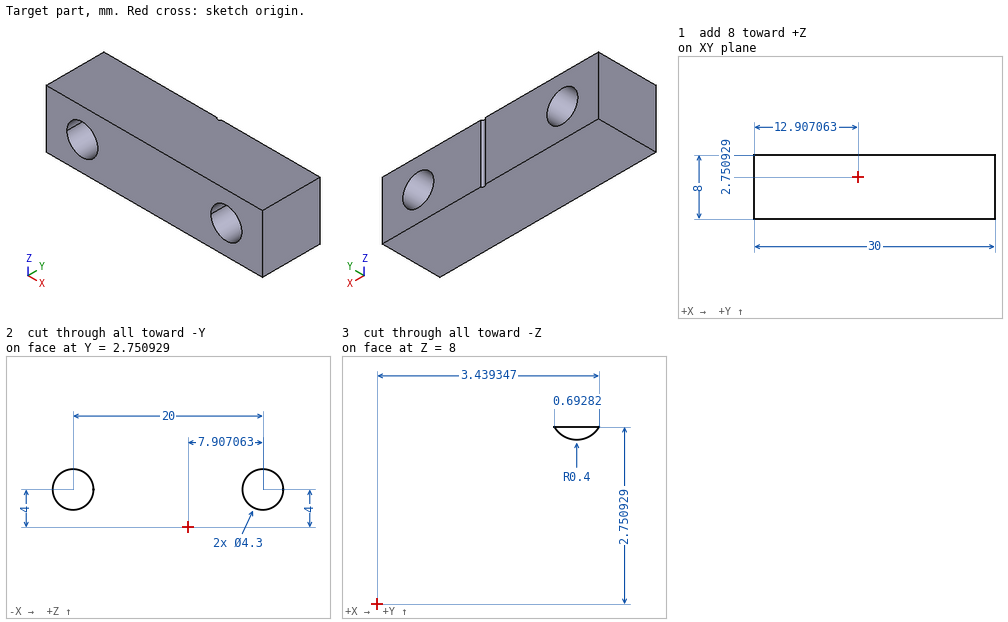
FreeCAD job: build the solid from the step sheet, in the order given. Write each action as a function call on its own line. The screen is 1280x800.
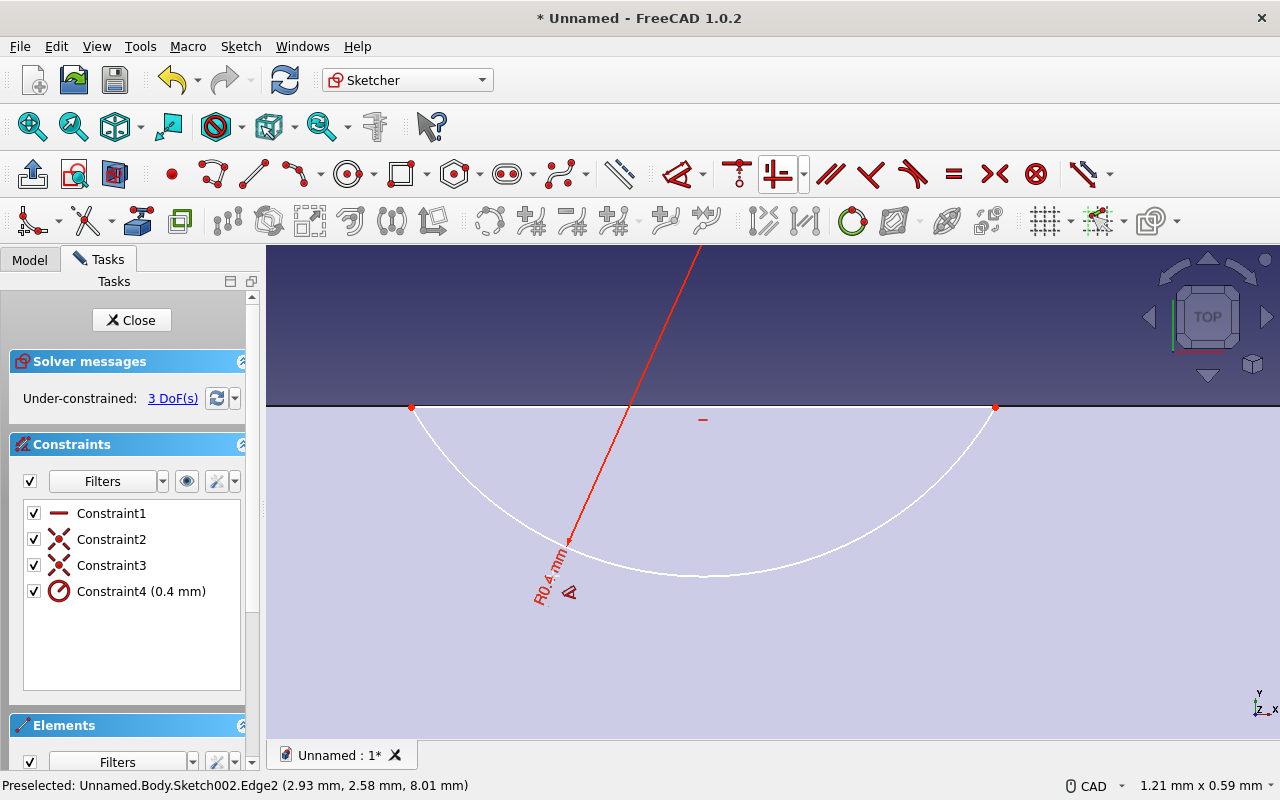
click(820, 407)
click(703, 373)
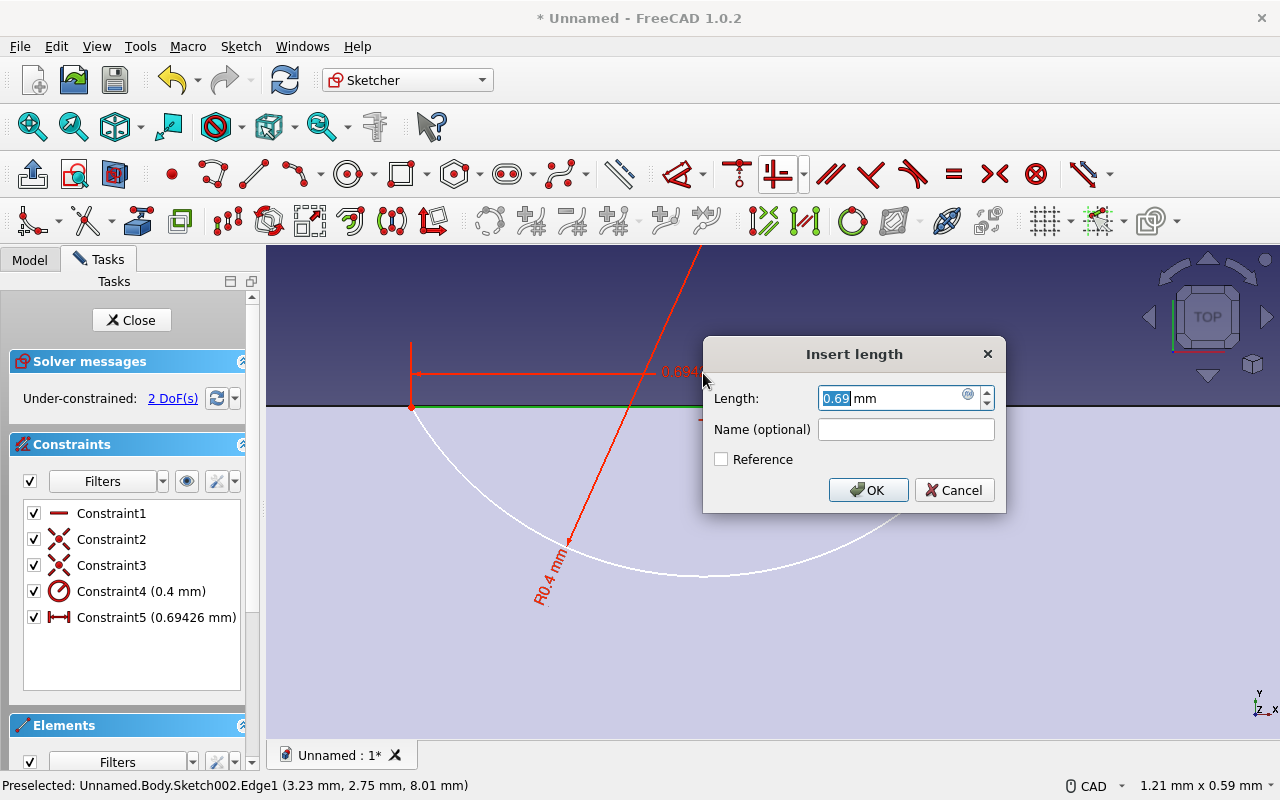
text(0.69282)
key(Return)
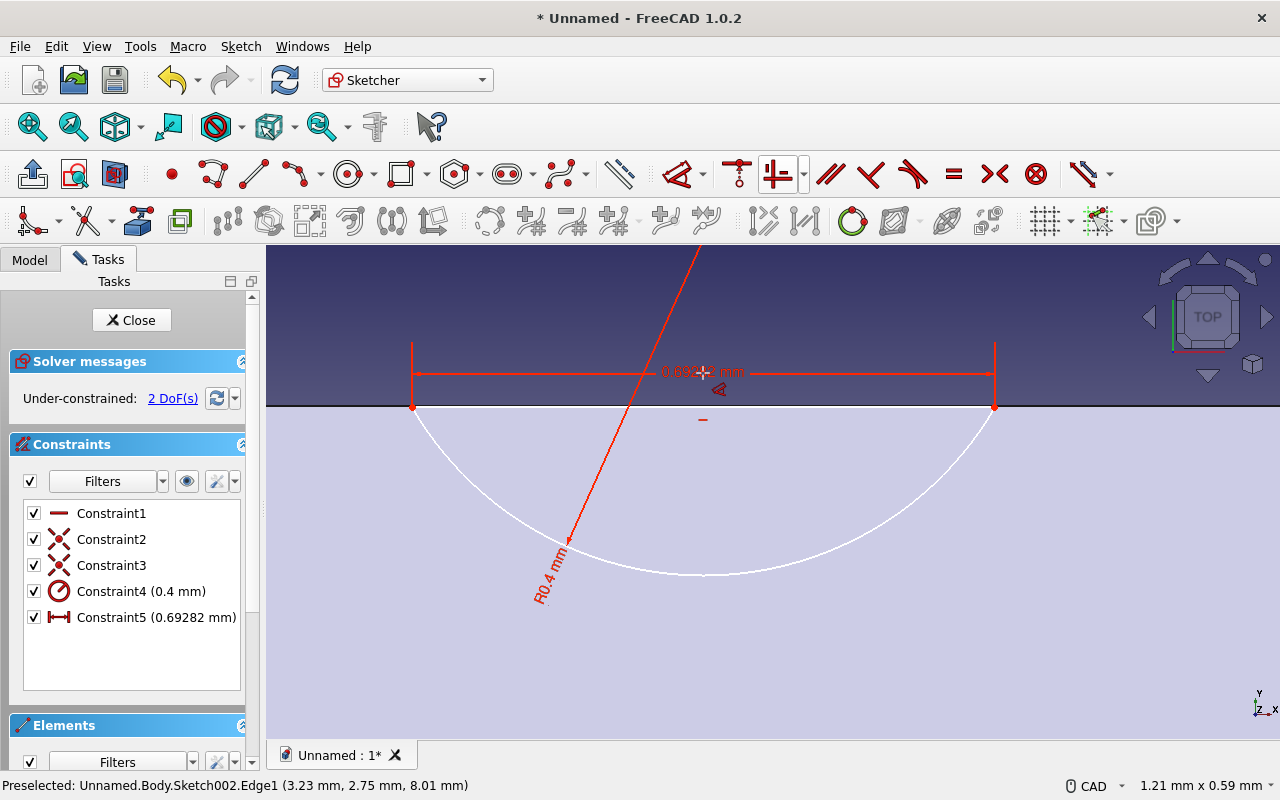
click(995, 407)
click(483, 373)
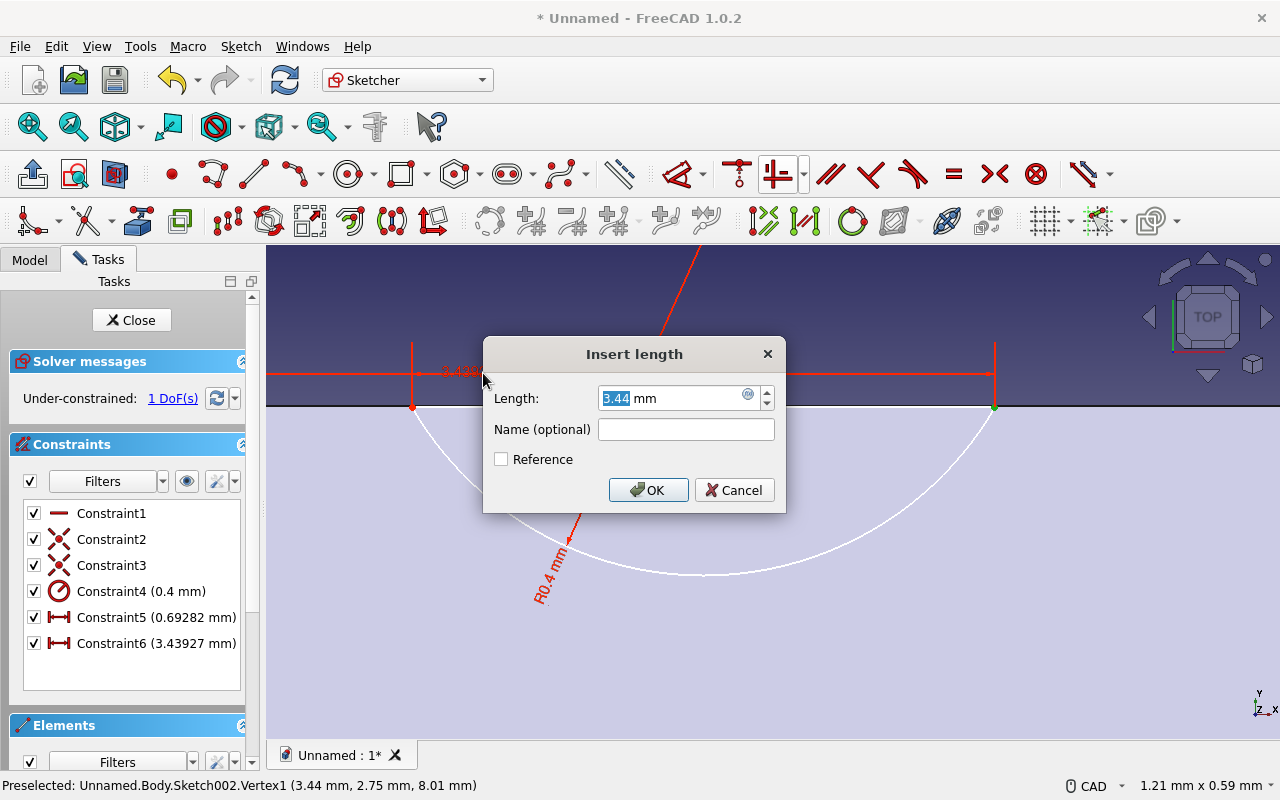
text(3.439347)
key(Return)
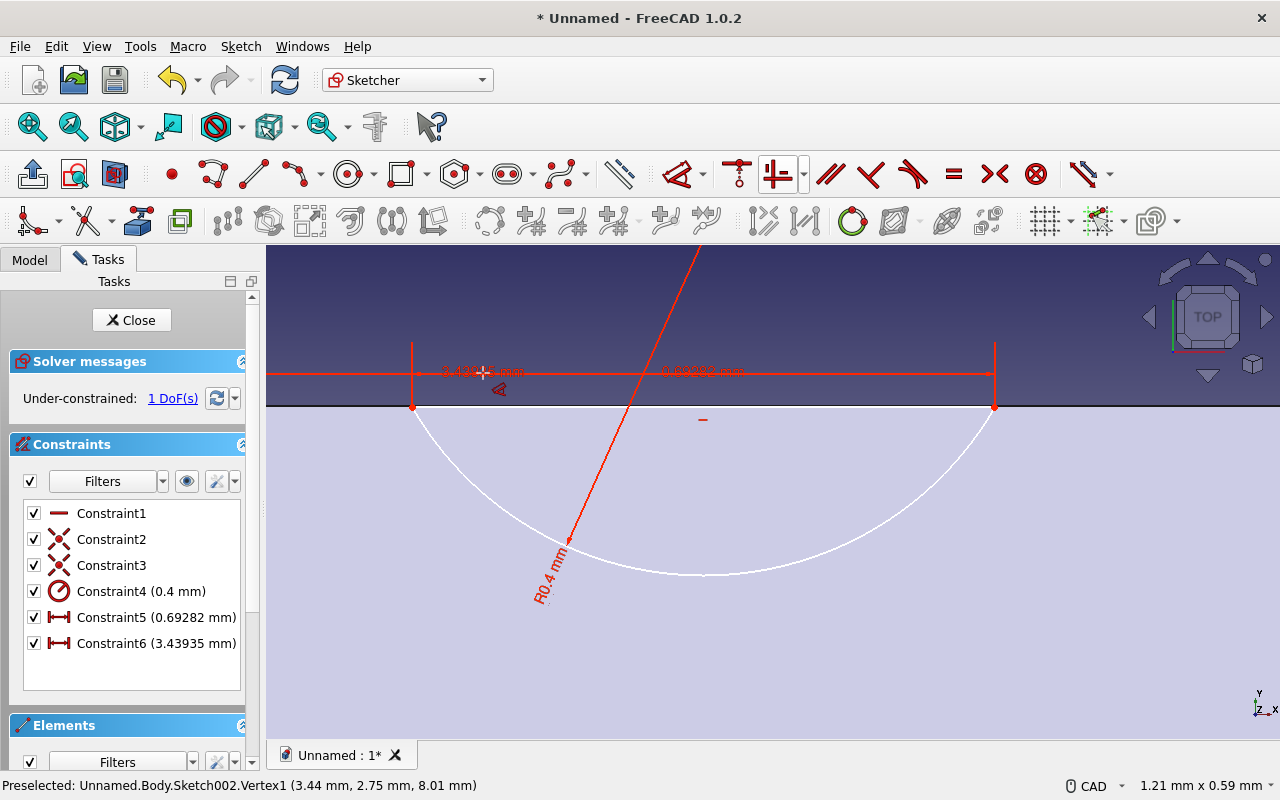
click(995, 407)
click(1029, 559)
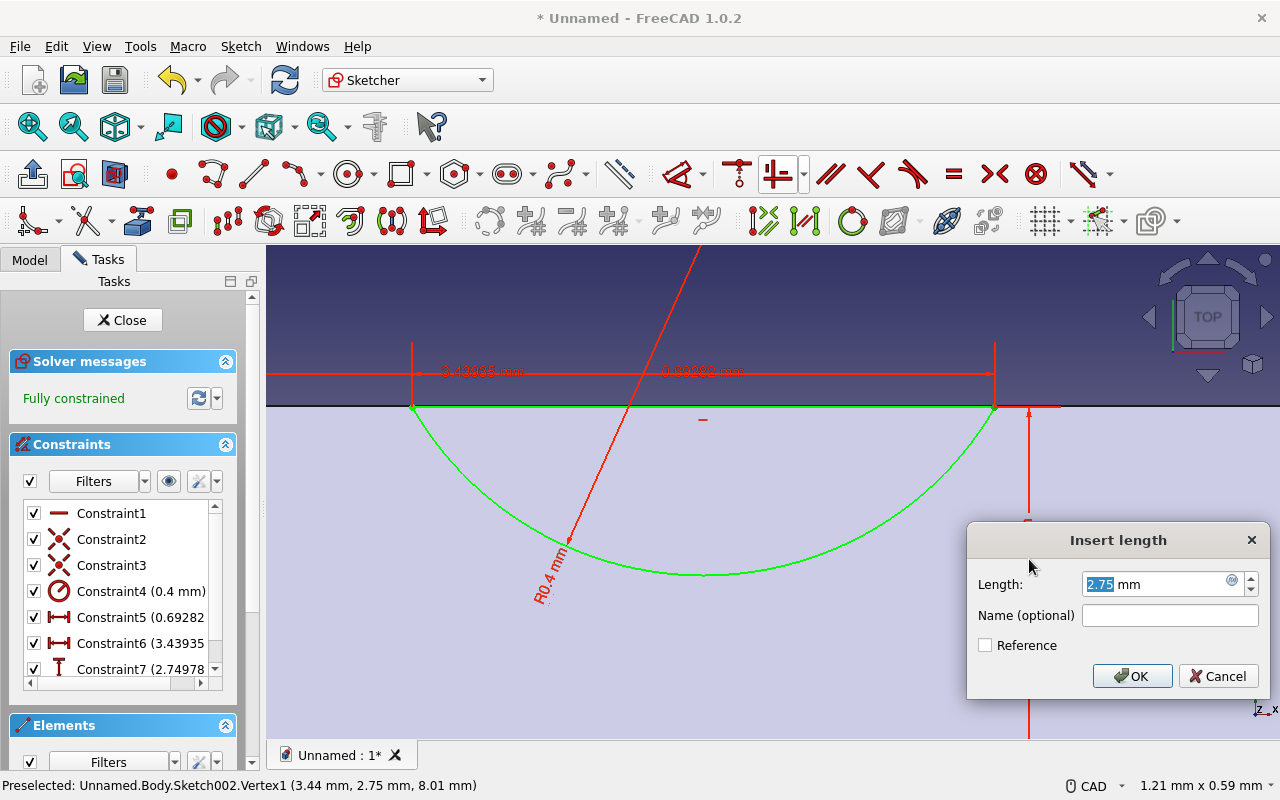
text(2.750929)
key(Return)
key(Escape)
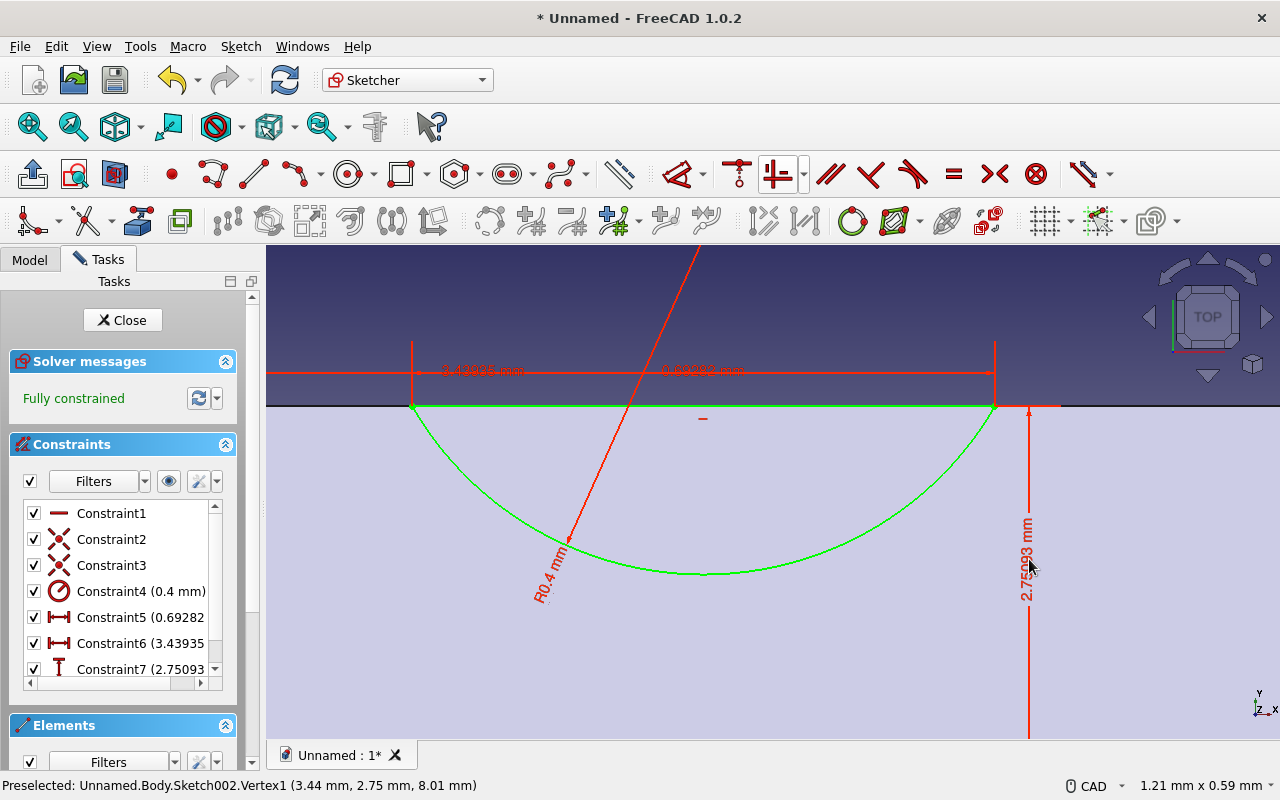
click(123, 320)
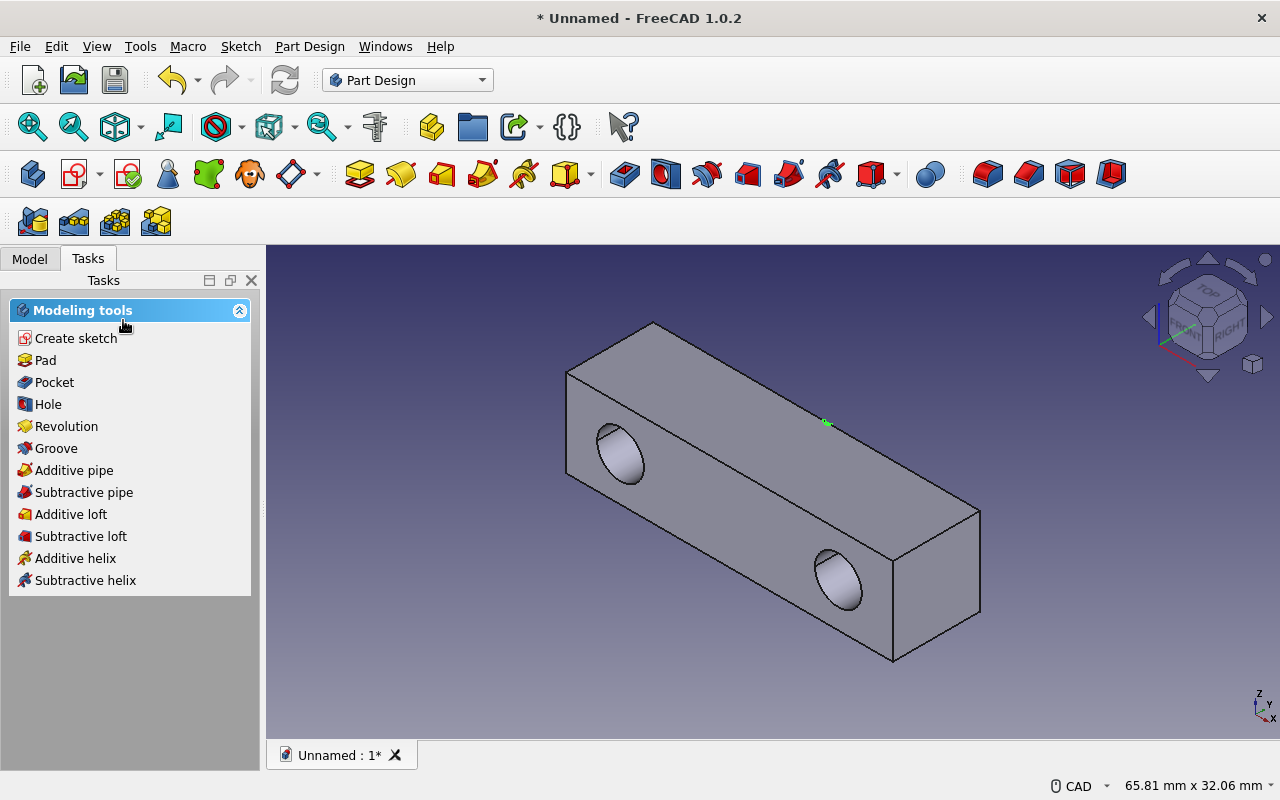
click(625, 174)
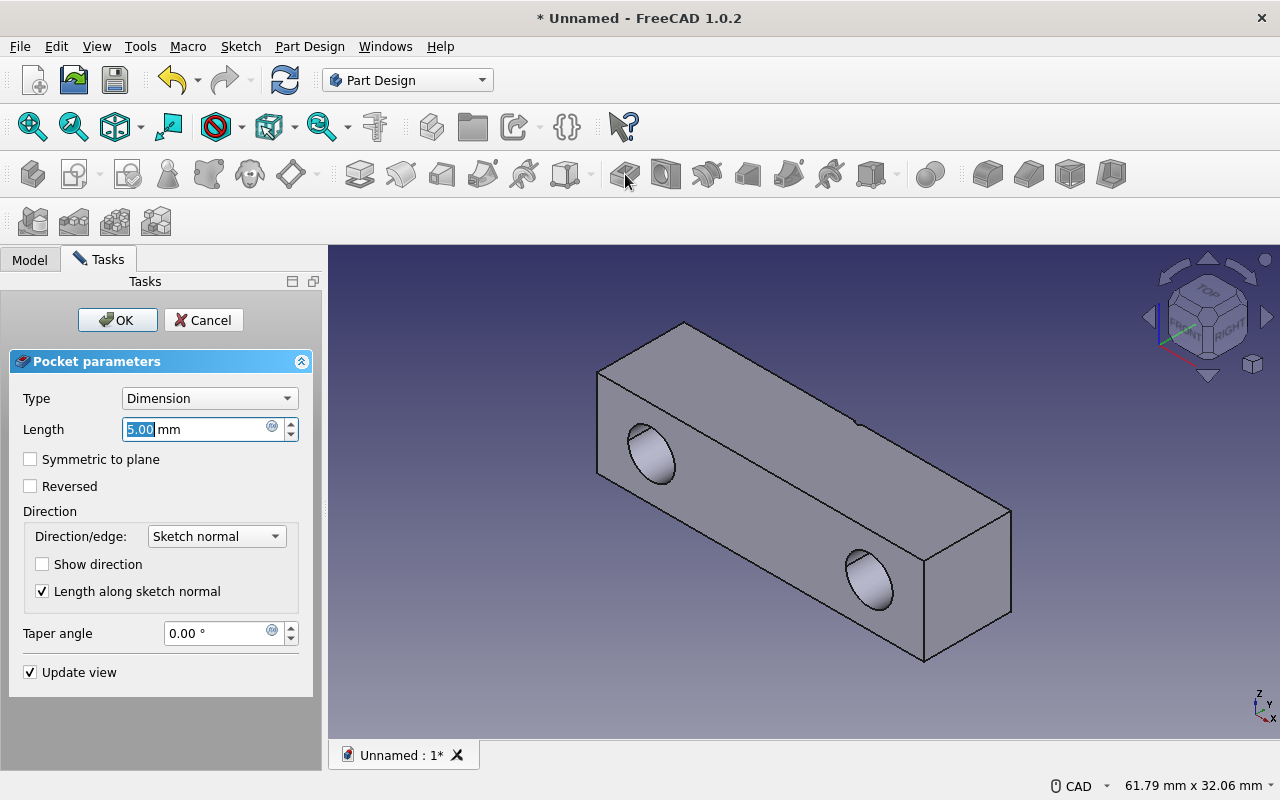
click(210, 398)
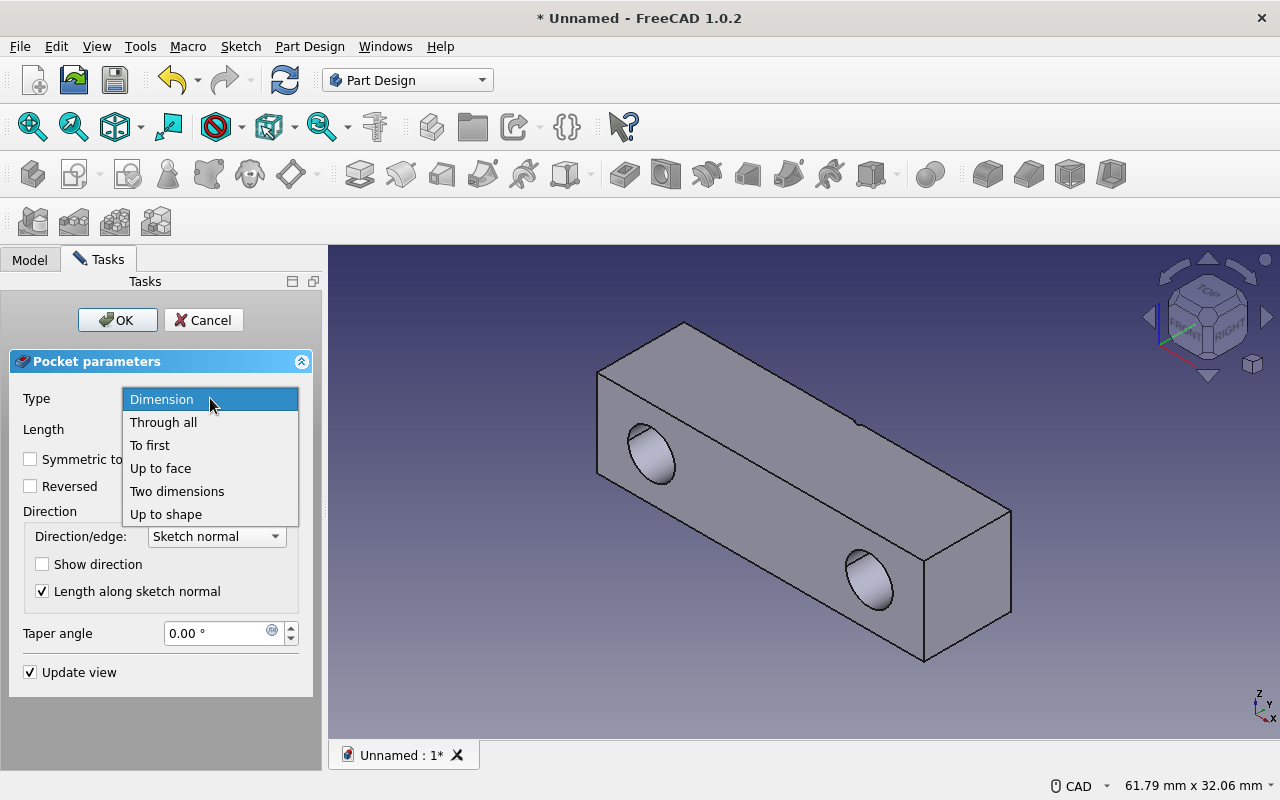
click(208, 422)